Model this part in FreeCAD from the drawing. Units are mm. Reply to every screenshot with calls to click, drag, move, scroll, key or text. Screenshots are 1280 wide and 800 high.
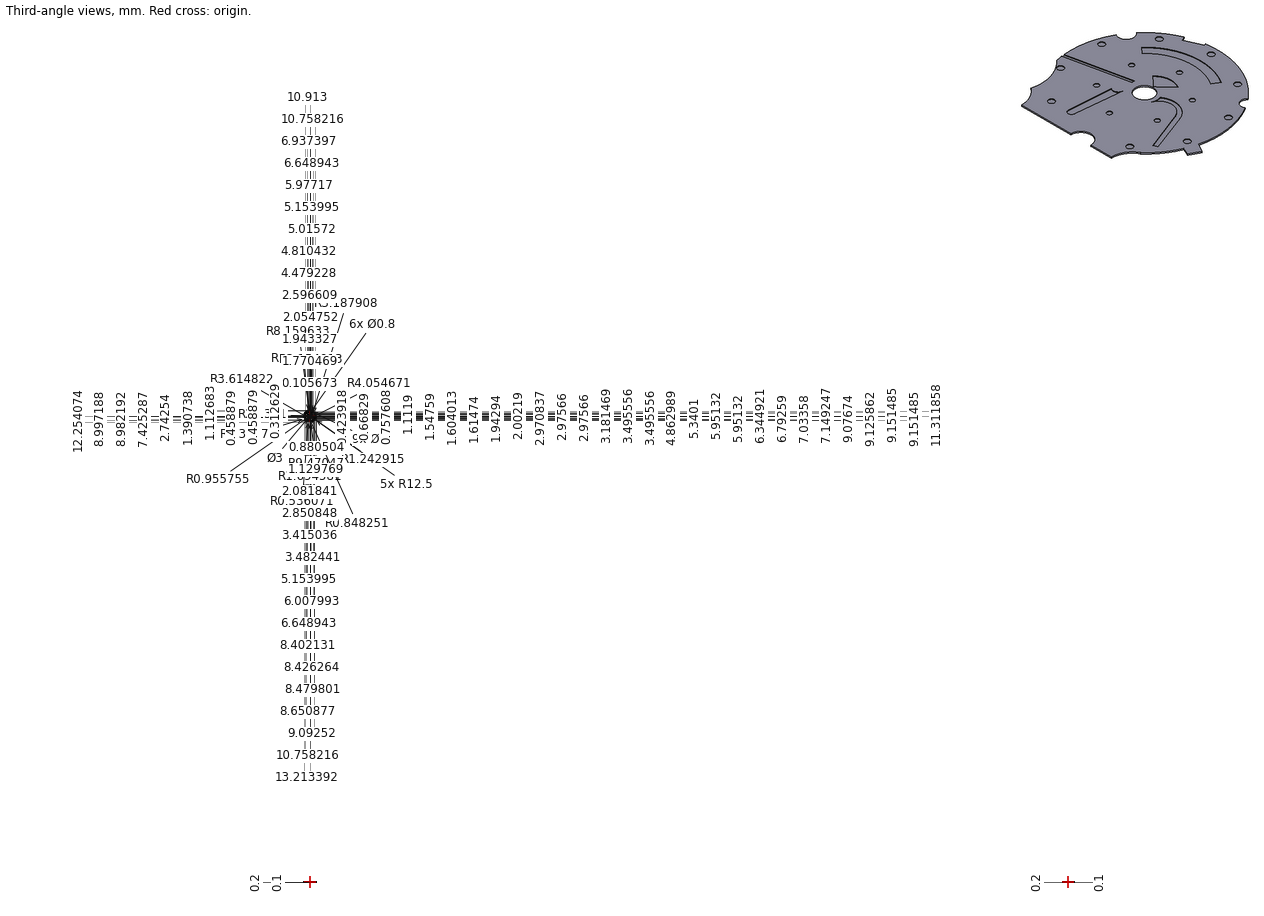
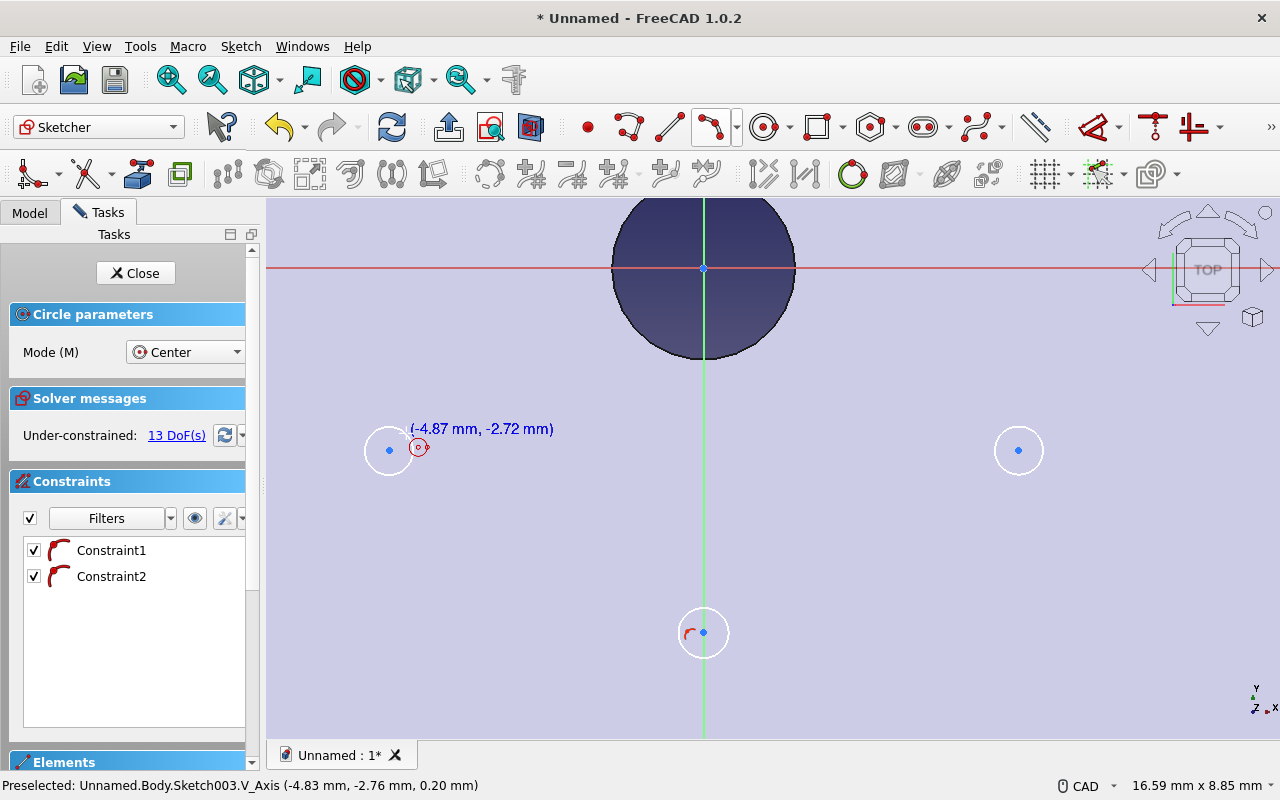
scroll(705, 632, down, 4)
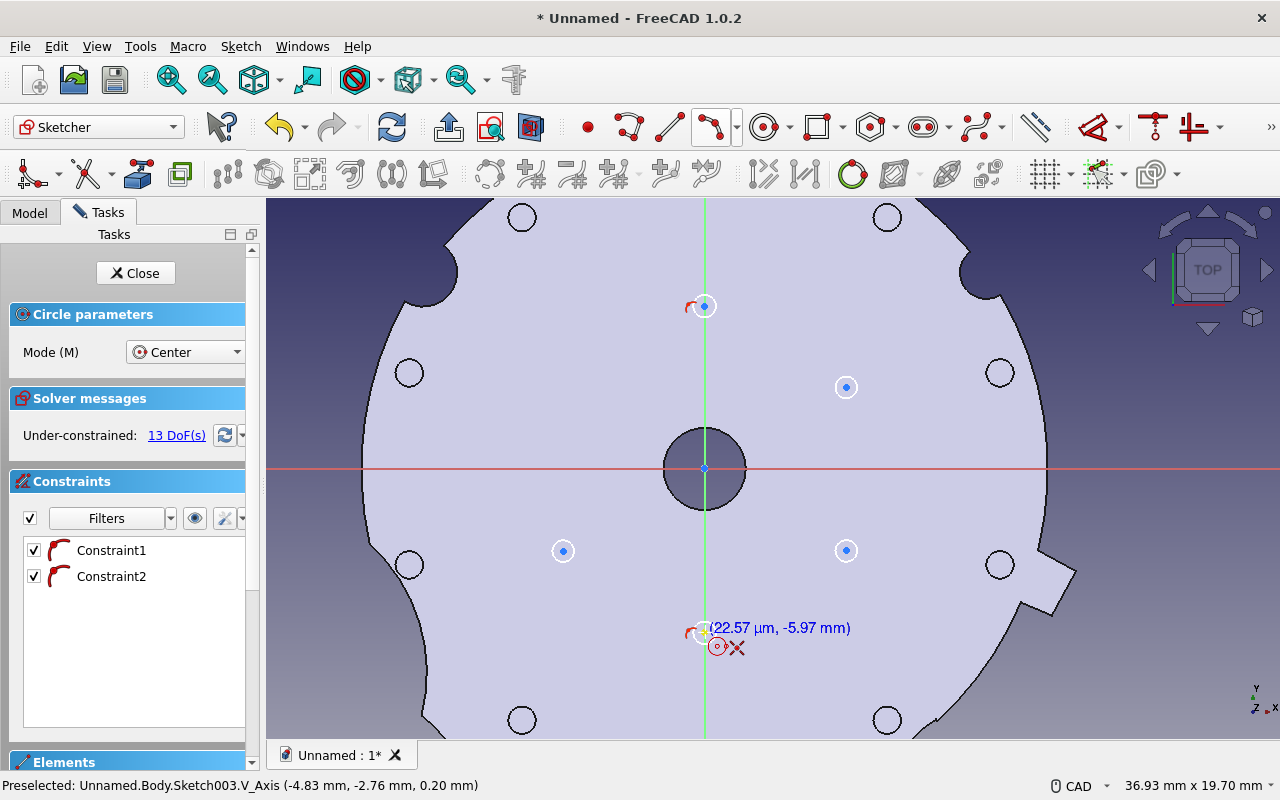
scroll(563, 387, up, 4)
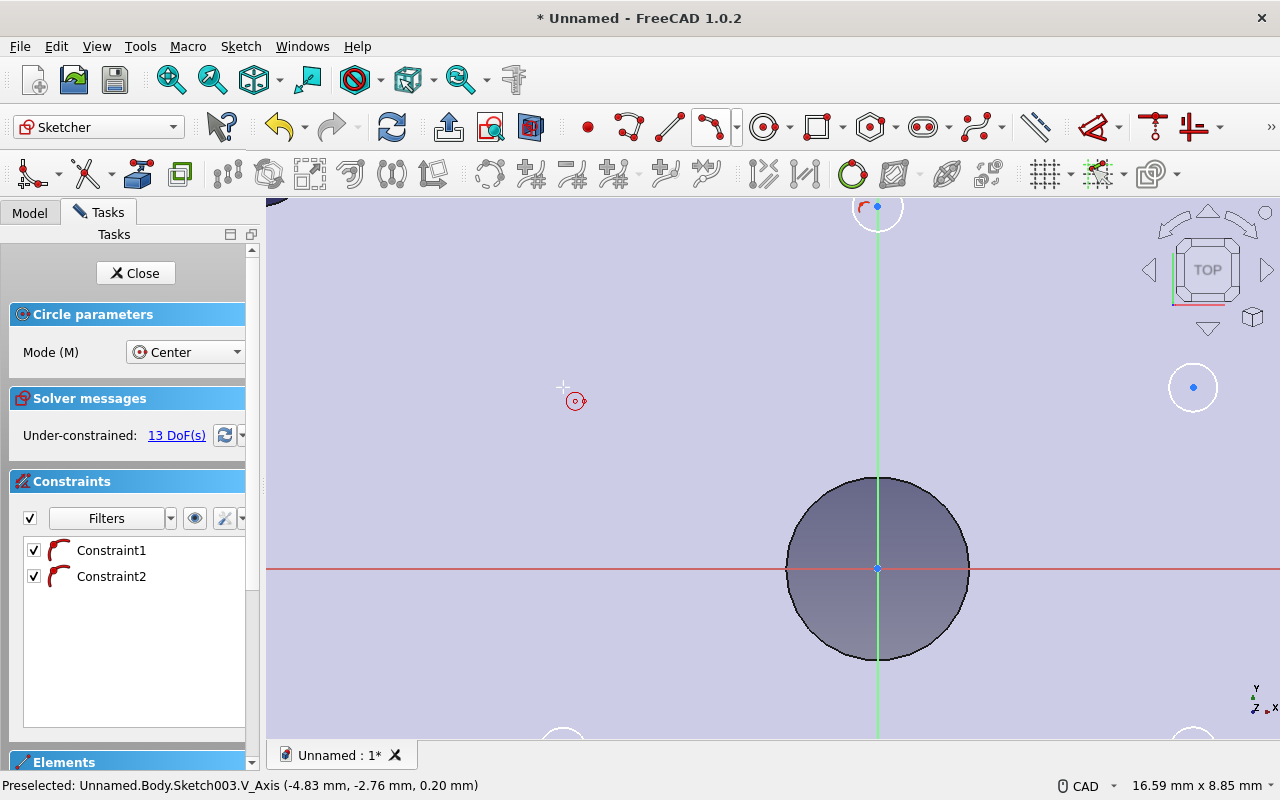
click(563, 387)
click(580, 370)
key(Escape)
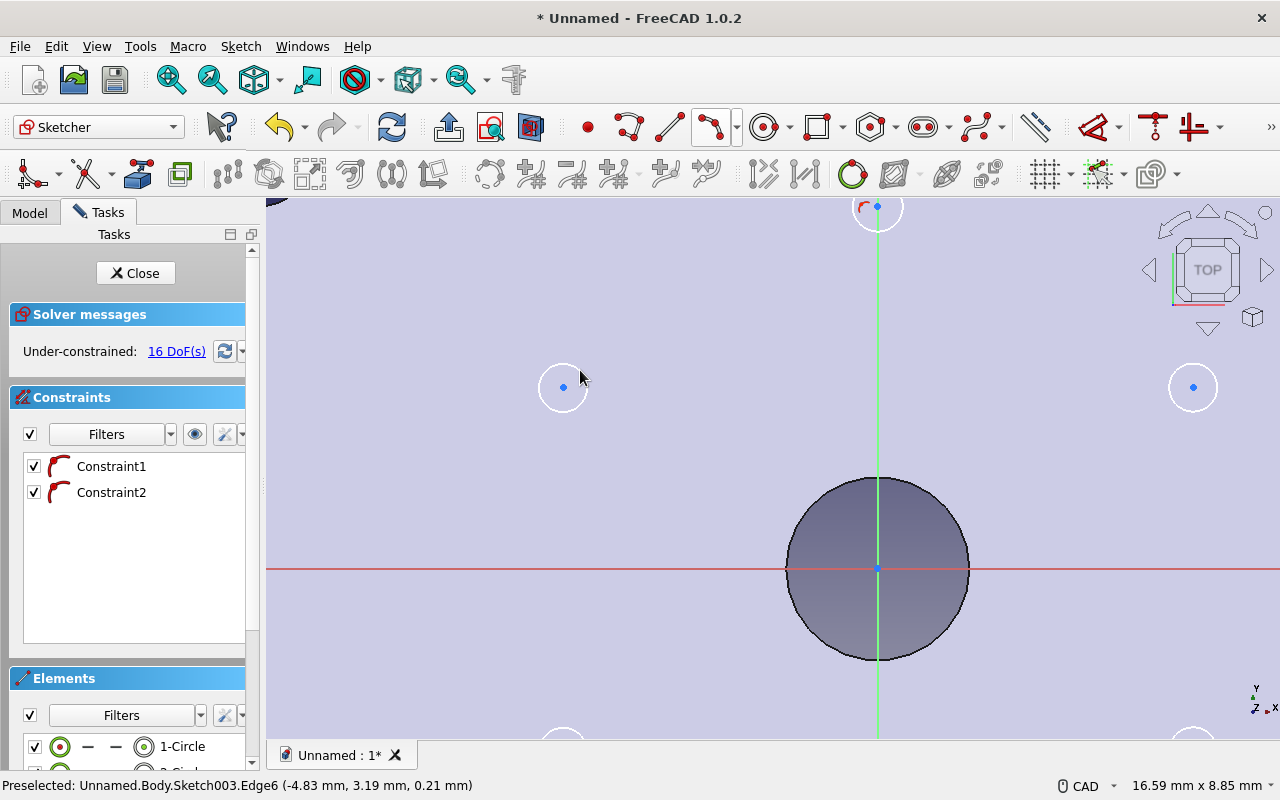
click(877, 232)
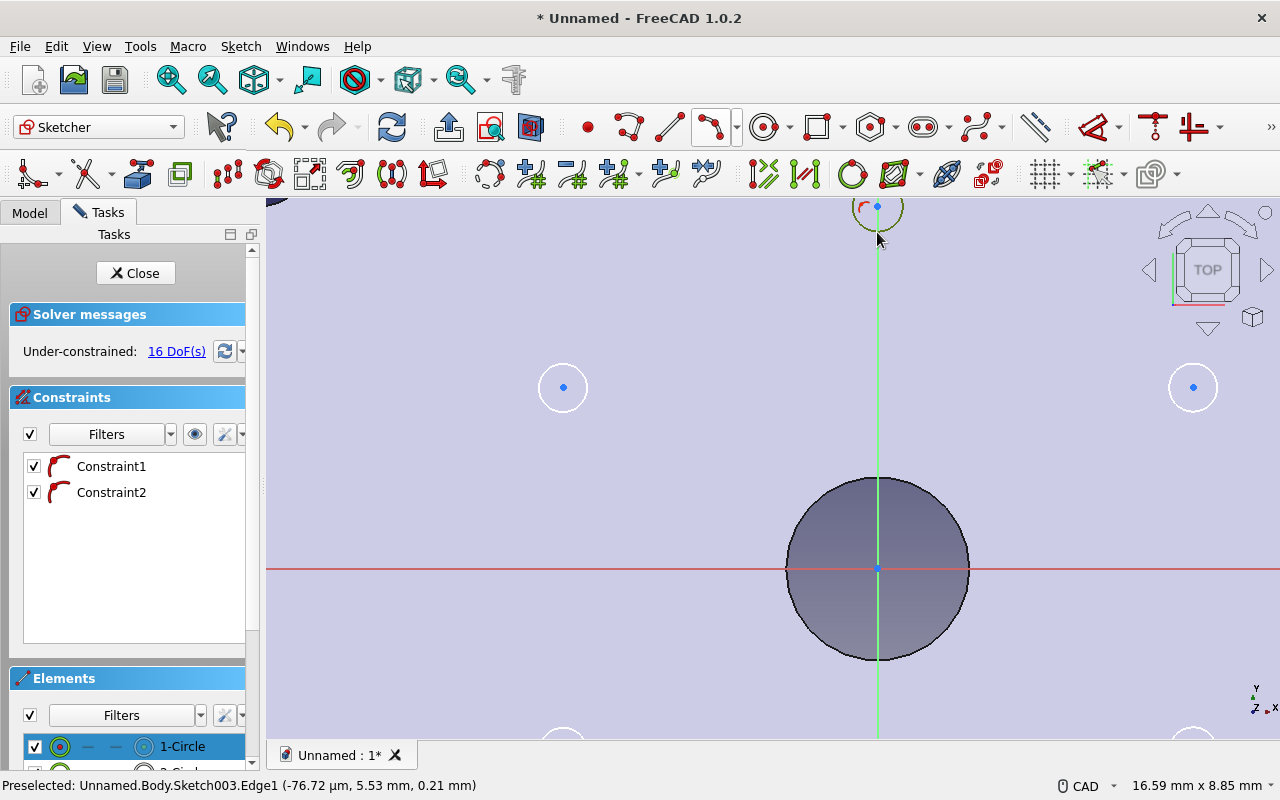
scroll(563, 387, down, 4)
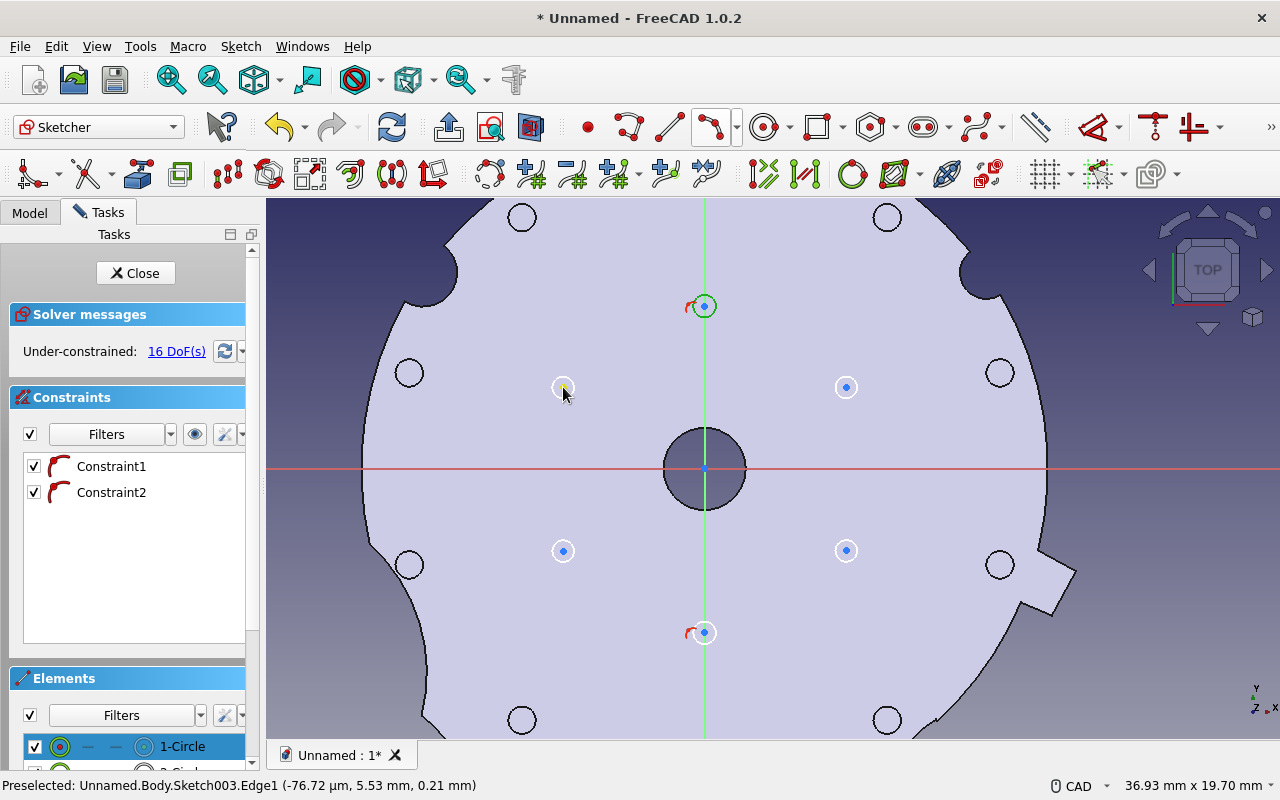
scroll(854, 380, up, 2)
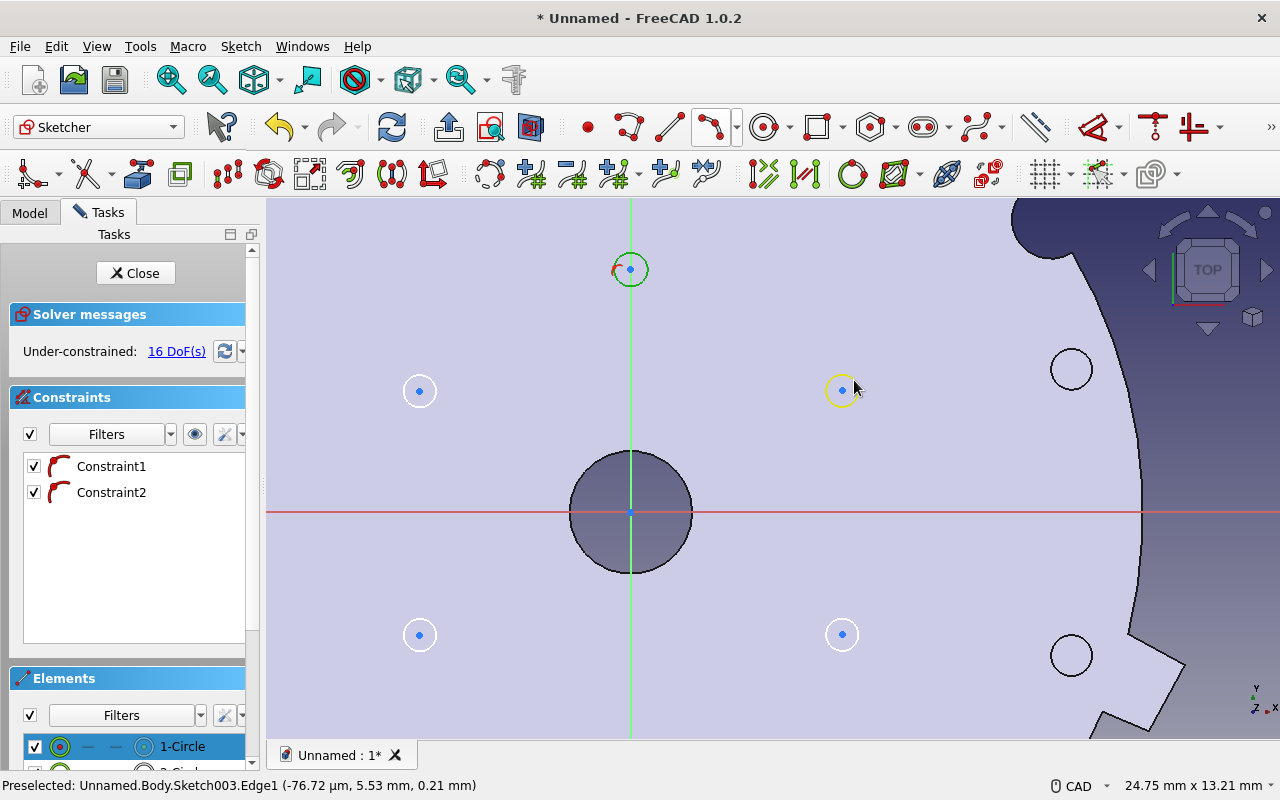
click(854, 380)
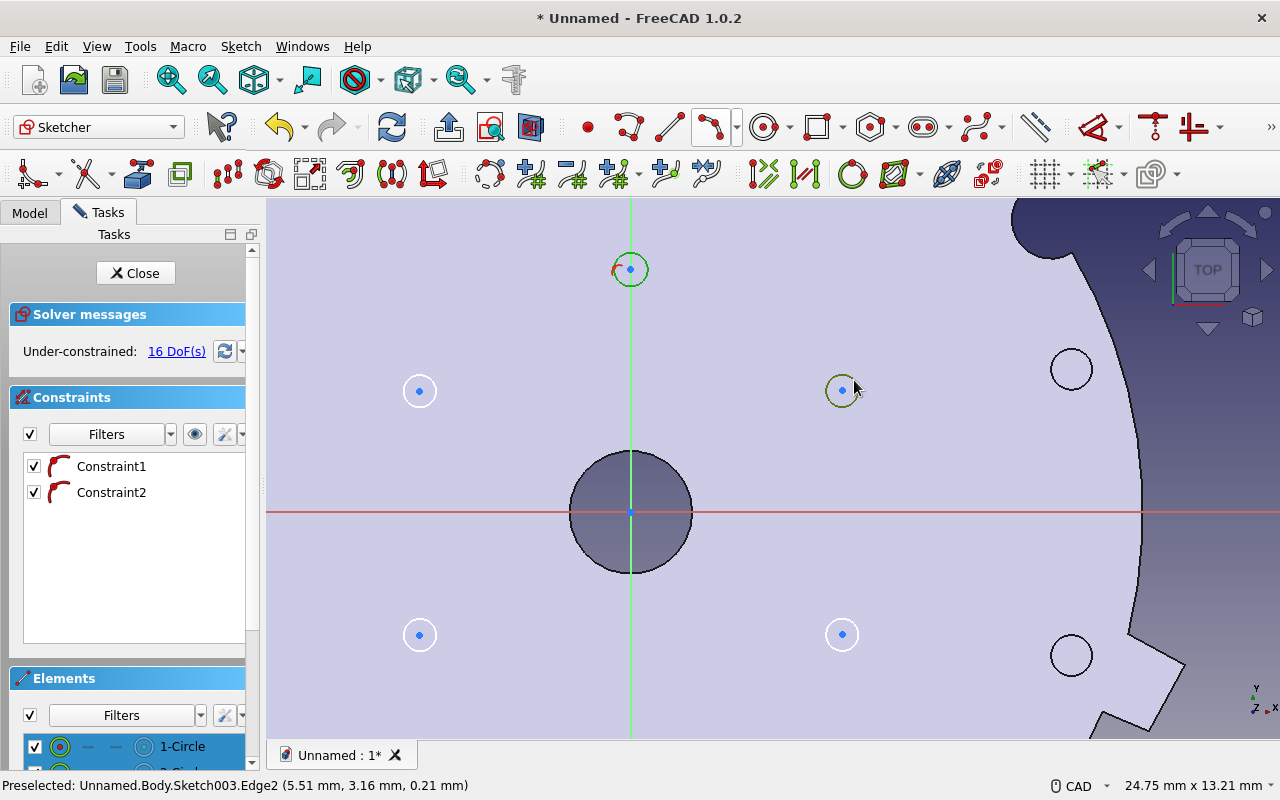
click(854, 623)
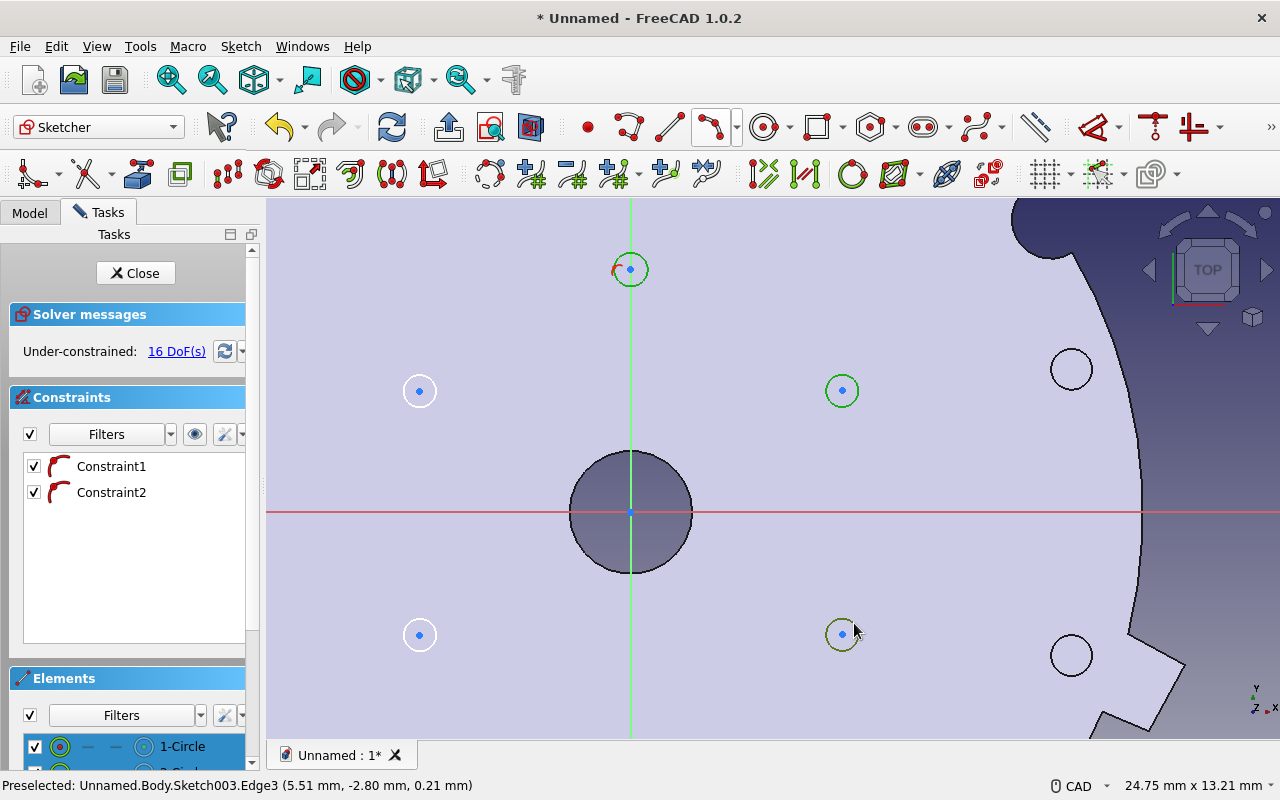
scroll(854, 379, down, 2)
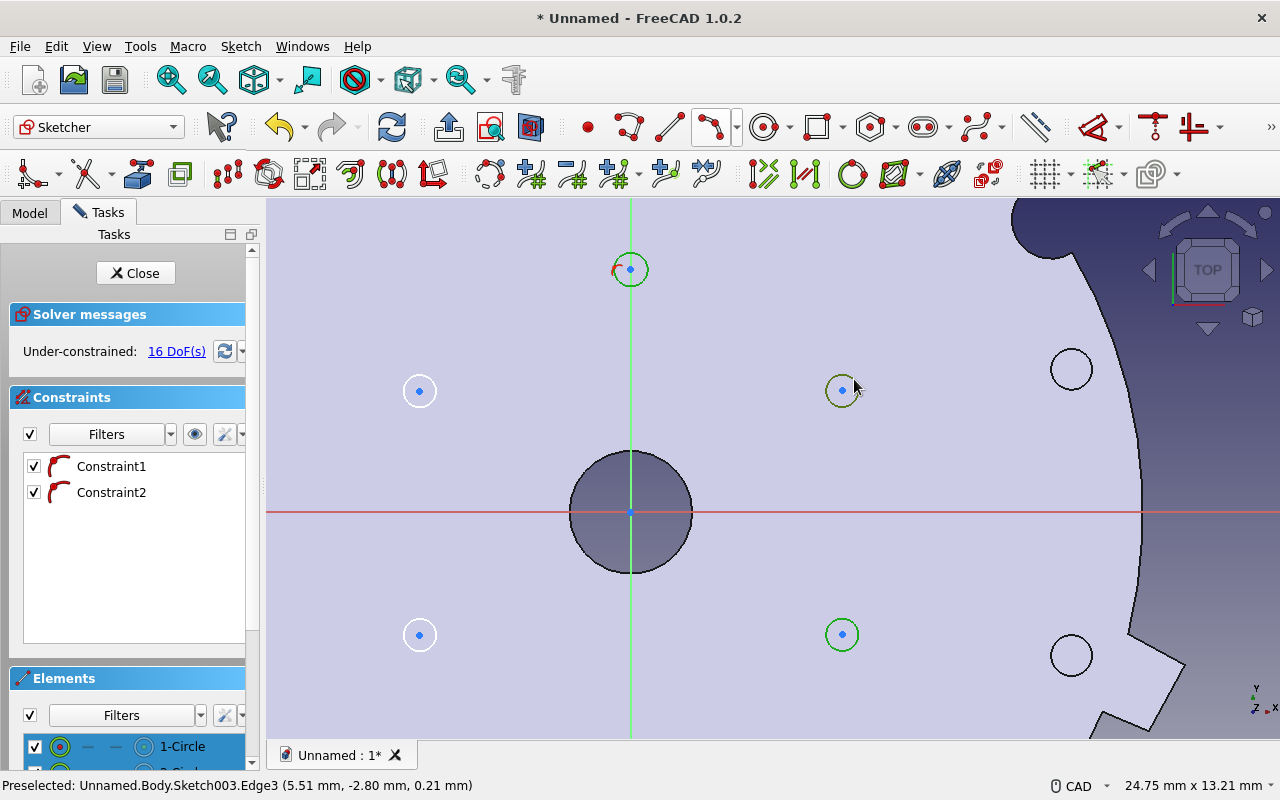
scroll(713, 625, up, 3)